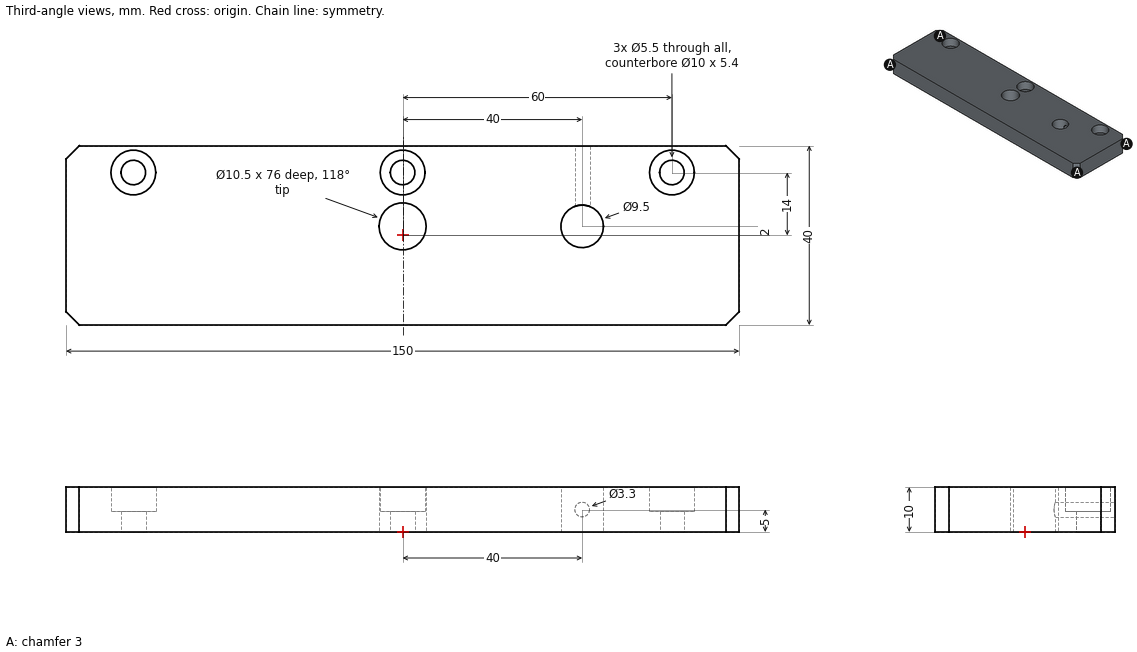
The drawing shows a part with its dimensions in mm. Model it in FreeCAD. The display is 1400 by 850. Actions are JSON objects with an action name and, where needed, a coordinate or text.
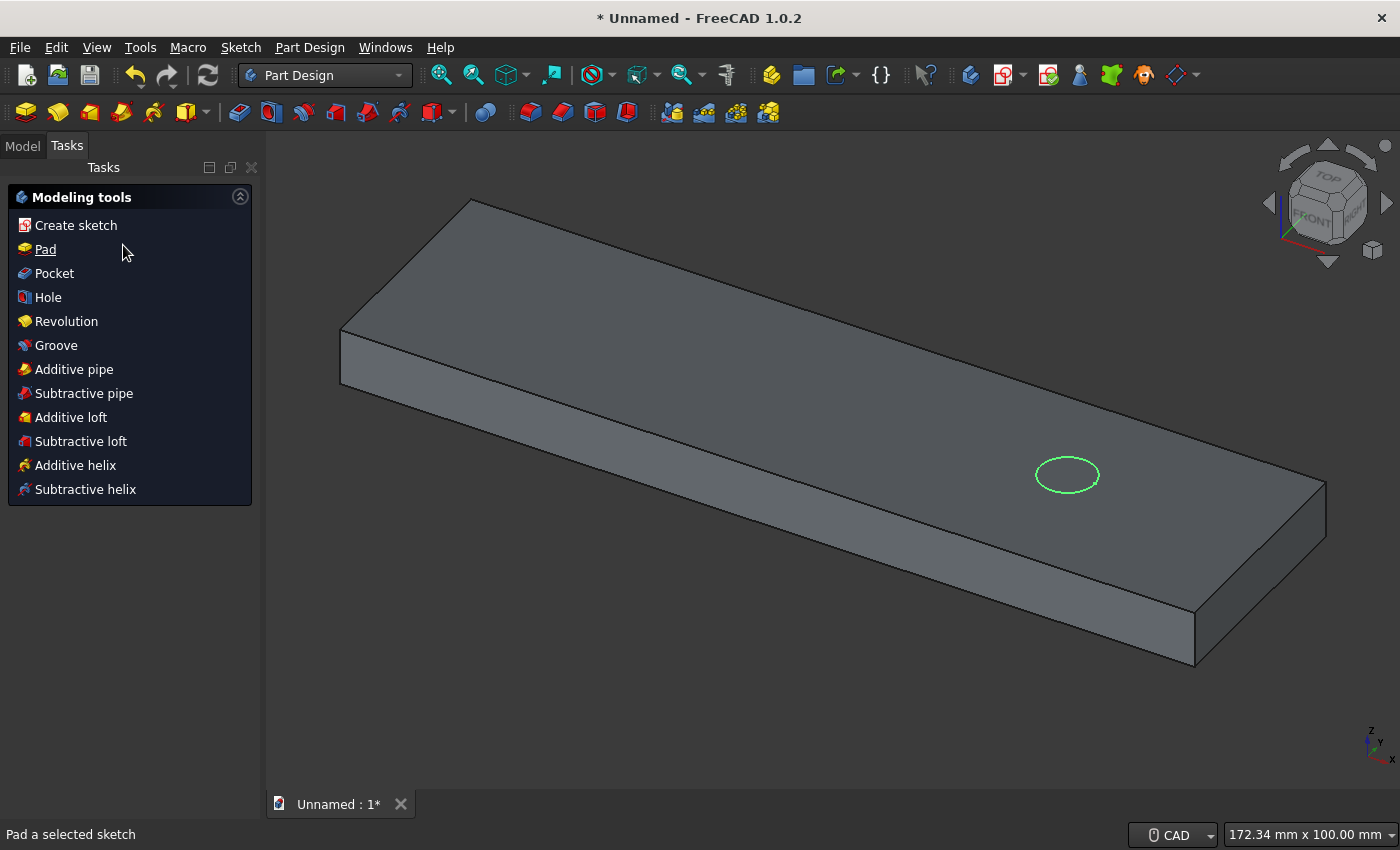
{"action": "left_click", "coordinate": [240, 112]}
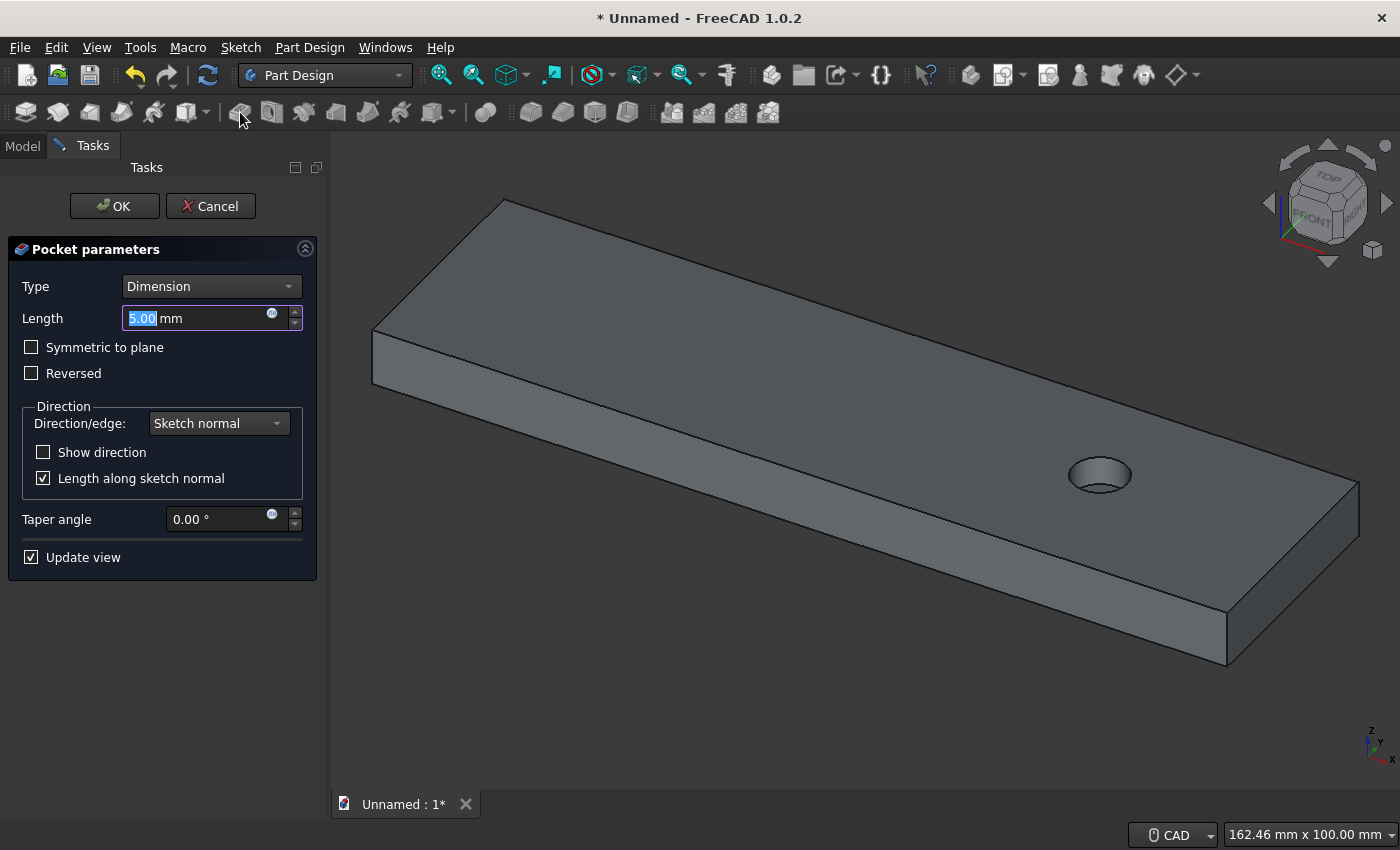
{"action": "left_click", "coordinate": [212, 286]}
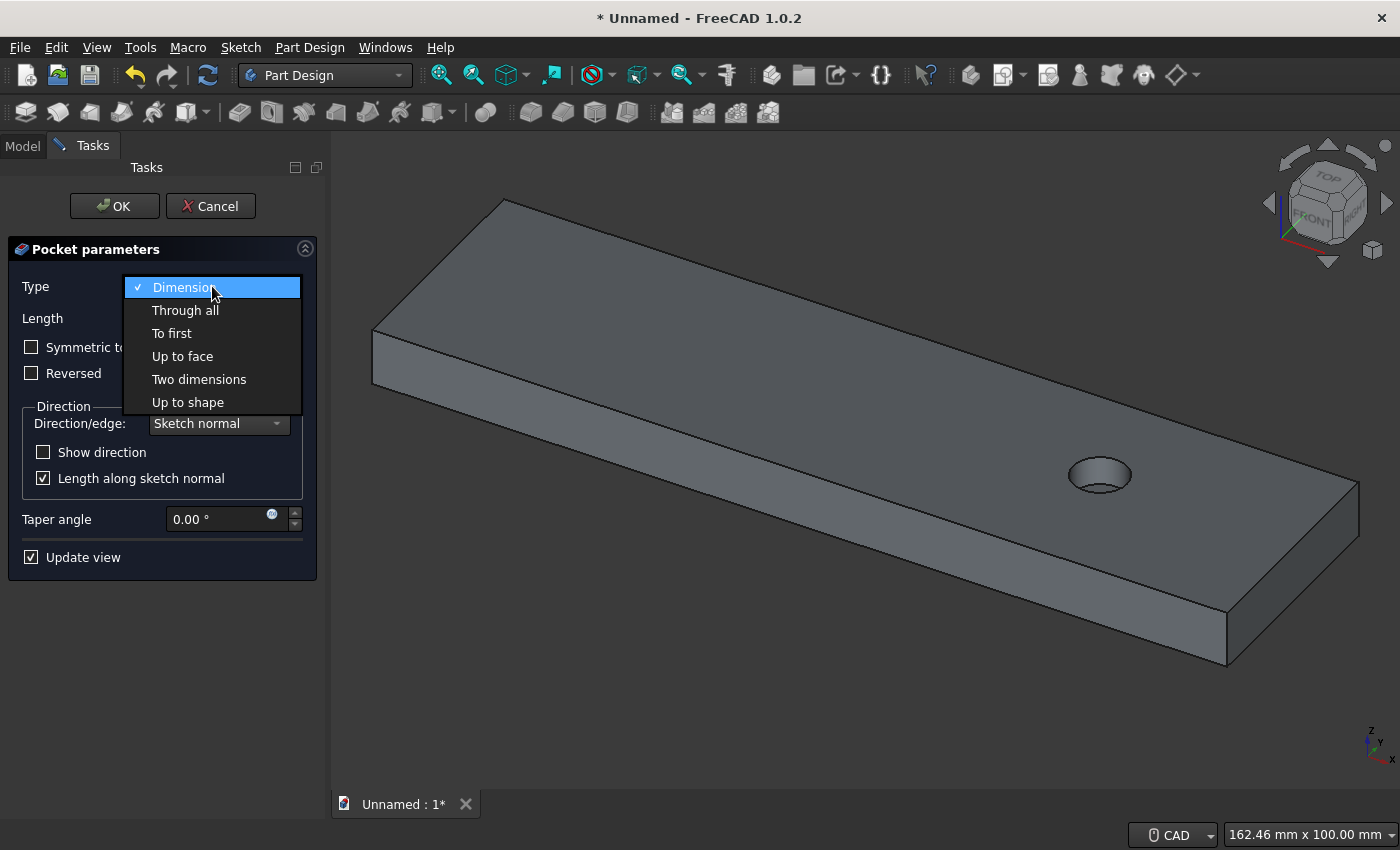
{"action": "left_click", "coordinate": [212, 310]}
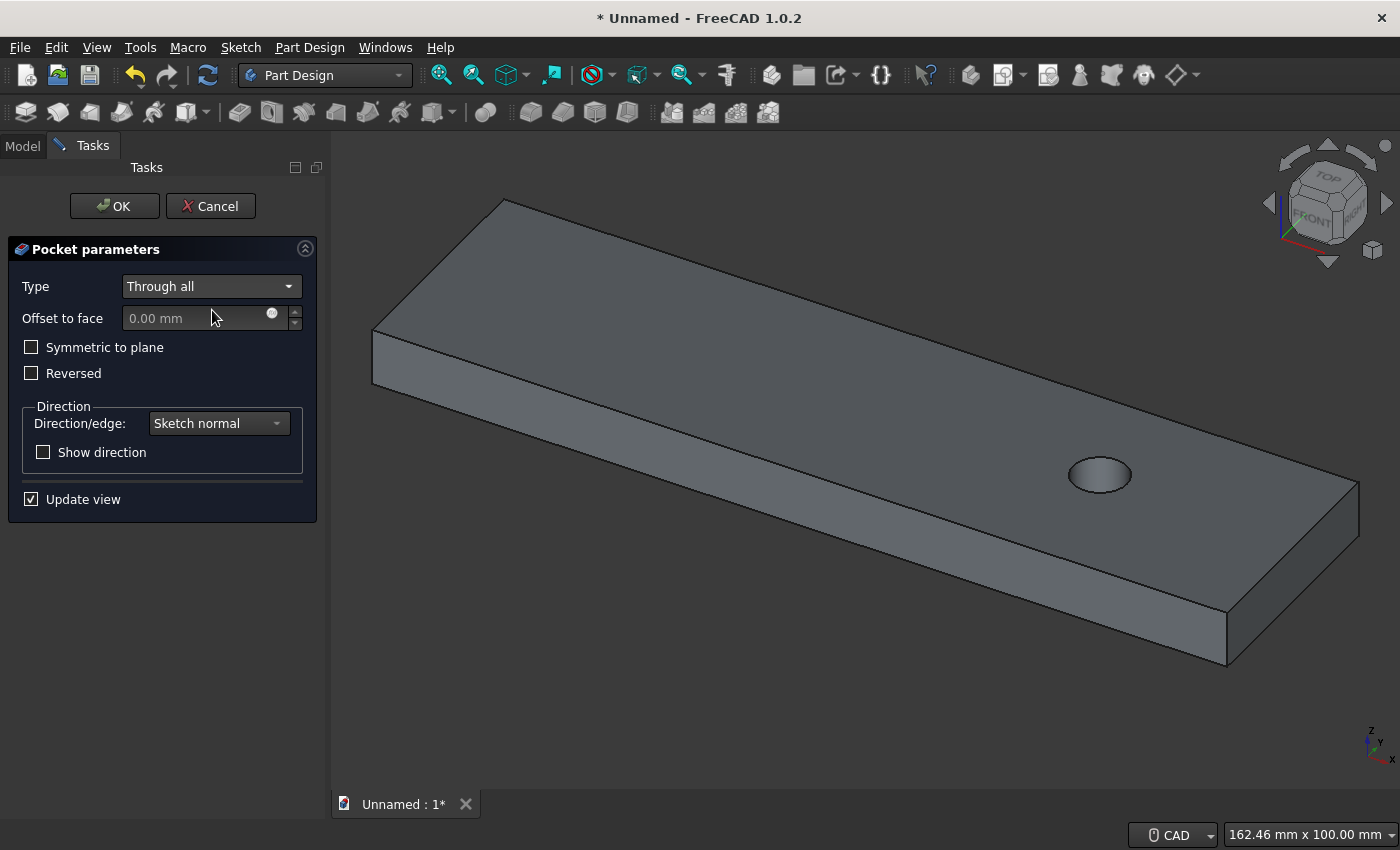
{"action": "left_click", "coordinate": [115, 206]}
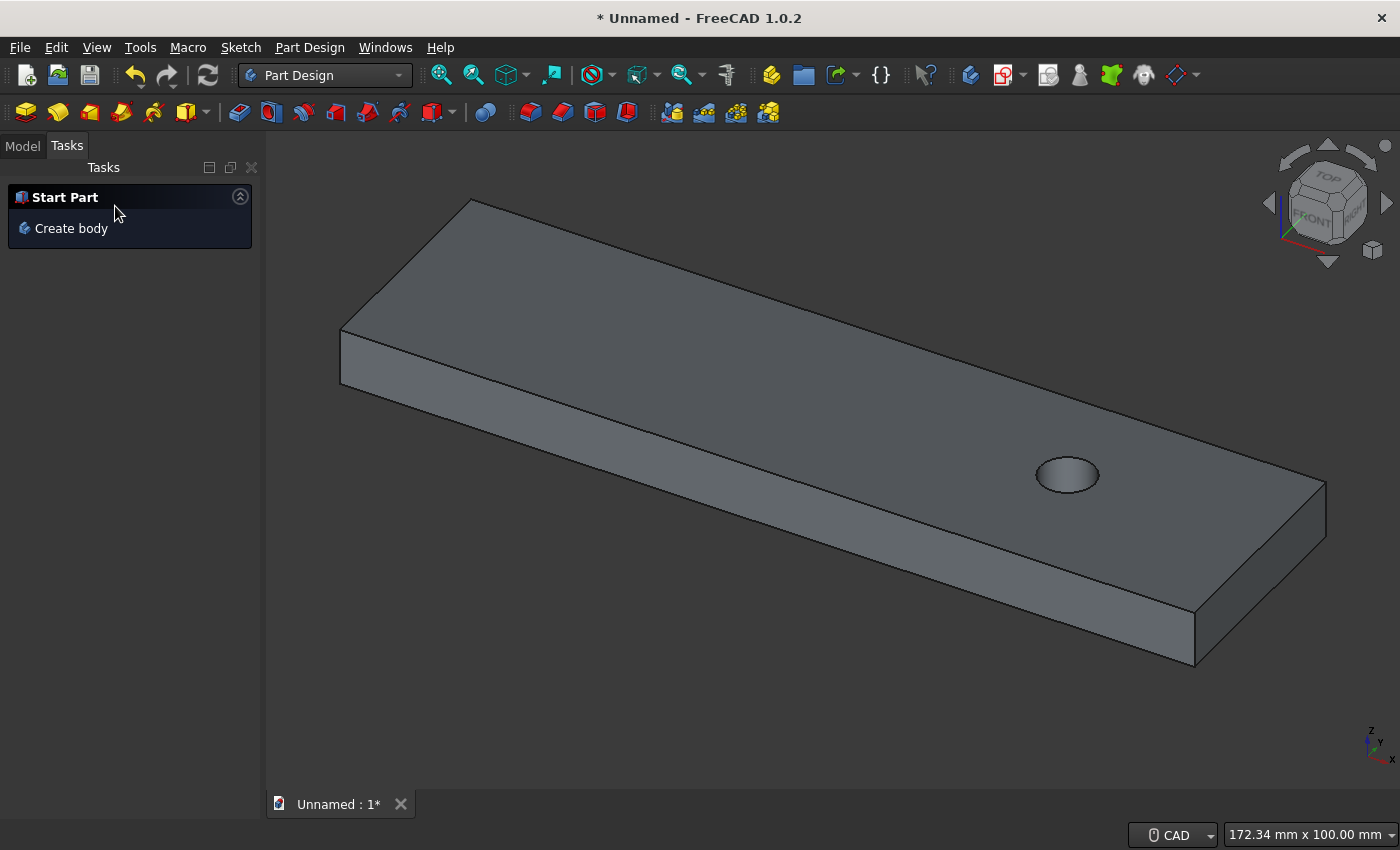
{"action": "left_click", "coordinate": [833, 405]}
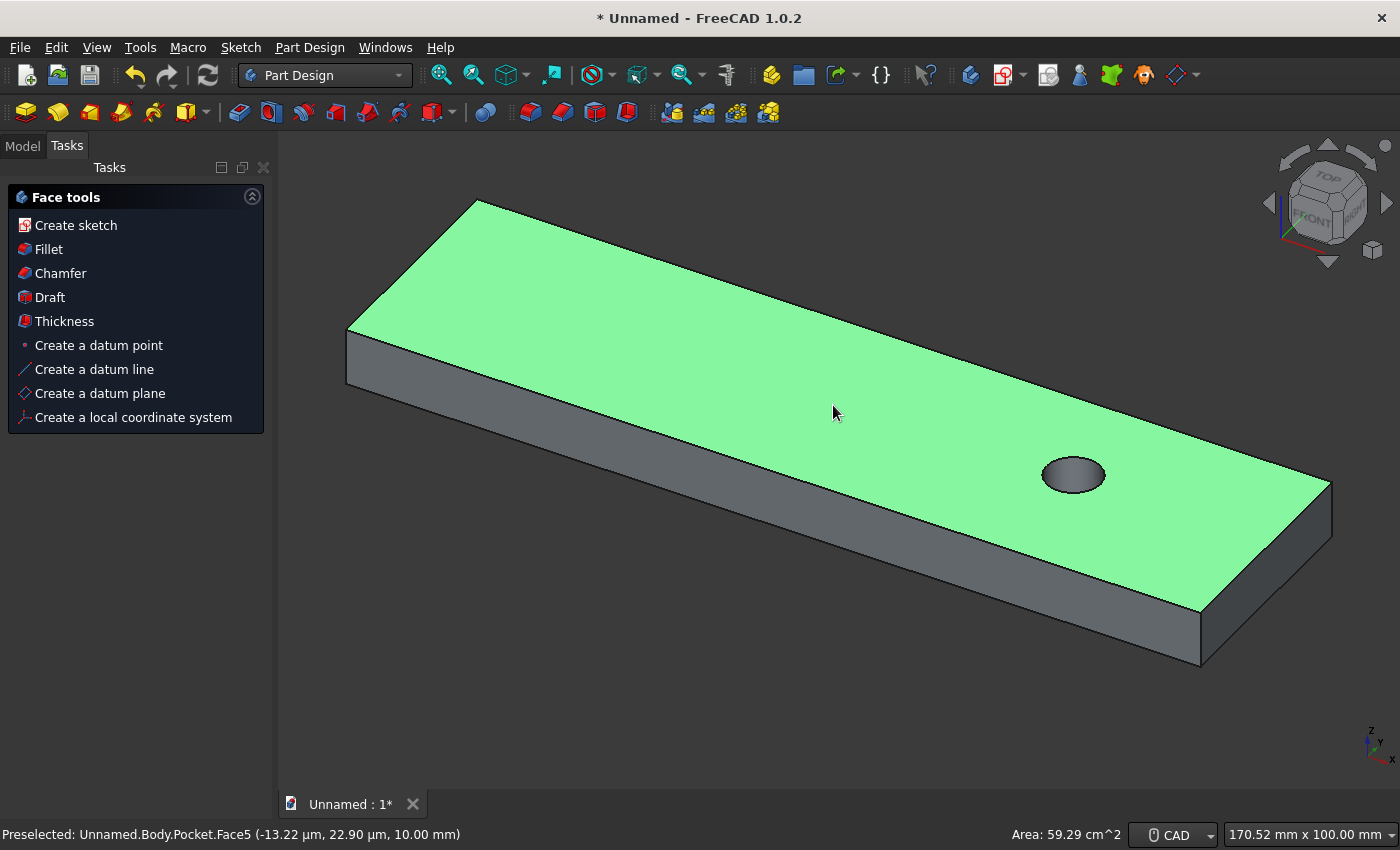
{"action": "left_click", "coordinate": [1004, 76]}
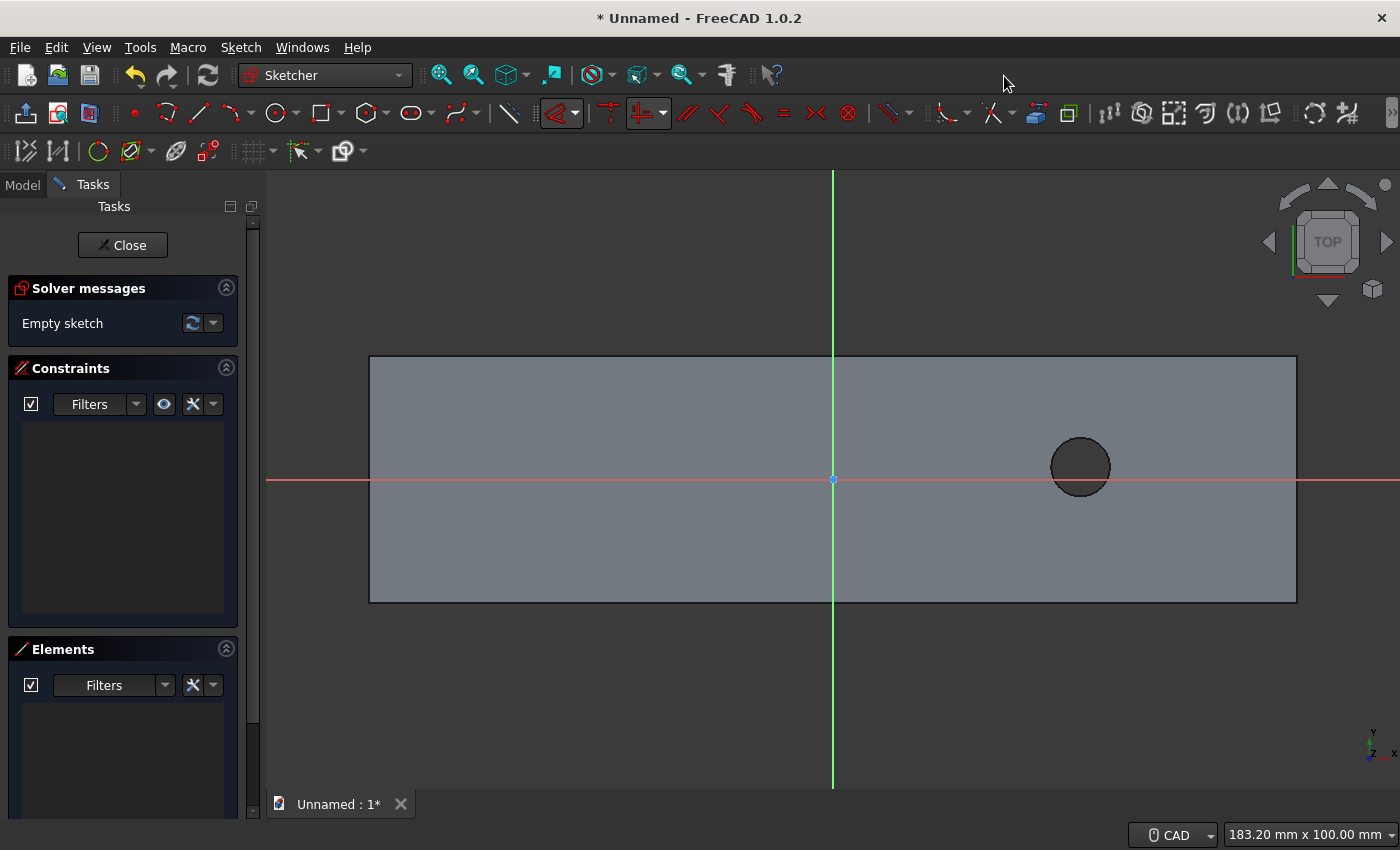
{"action": "scroll", "coordinate": [847, 465], "scroll_direction": "up", "scroll_amount": 9}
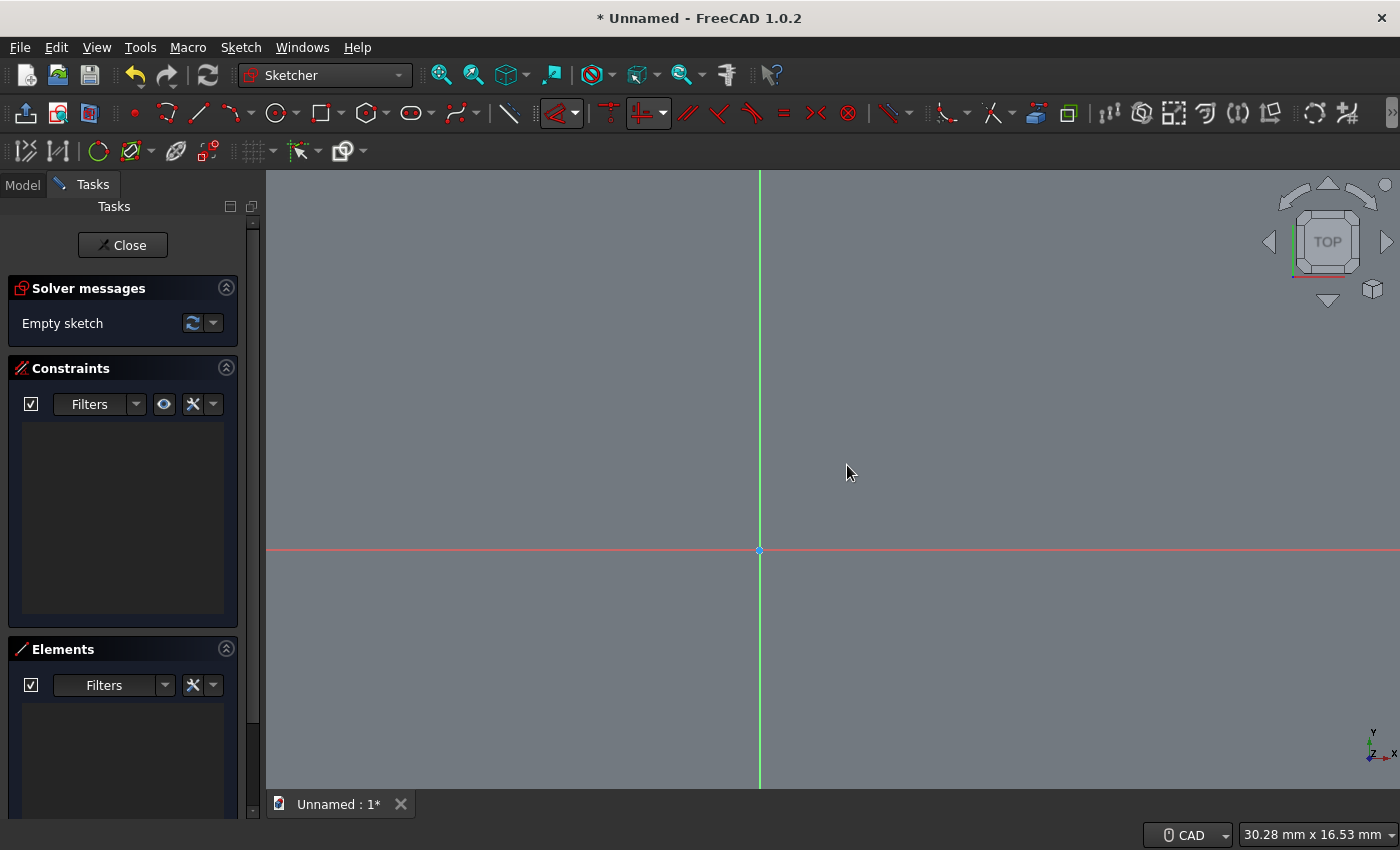
{"action": "key", "text": "g c"}